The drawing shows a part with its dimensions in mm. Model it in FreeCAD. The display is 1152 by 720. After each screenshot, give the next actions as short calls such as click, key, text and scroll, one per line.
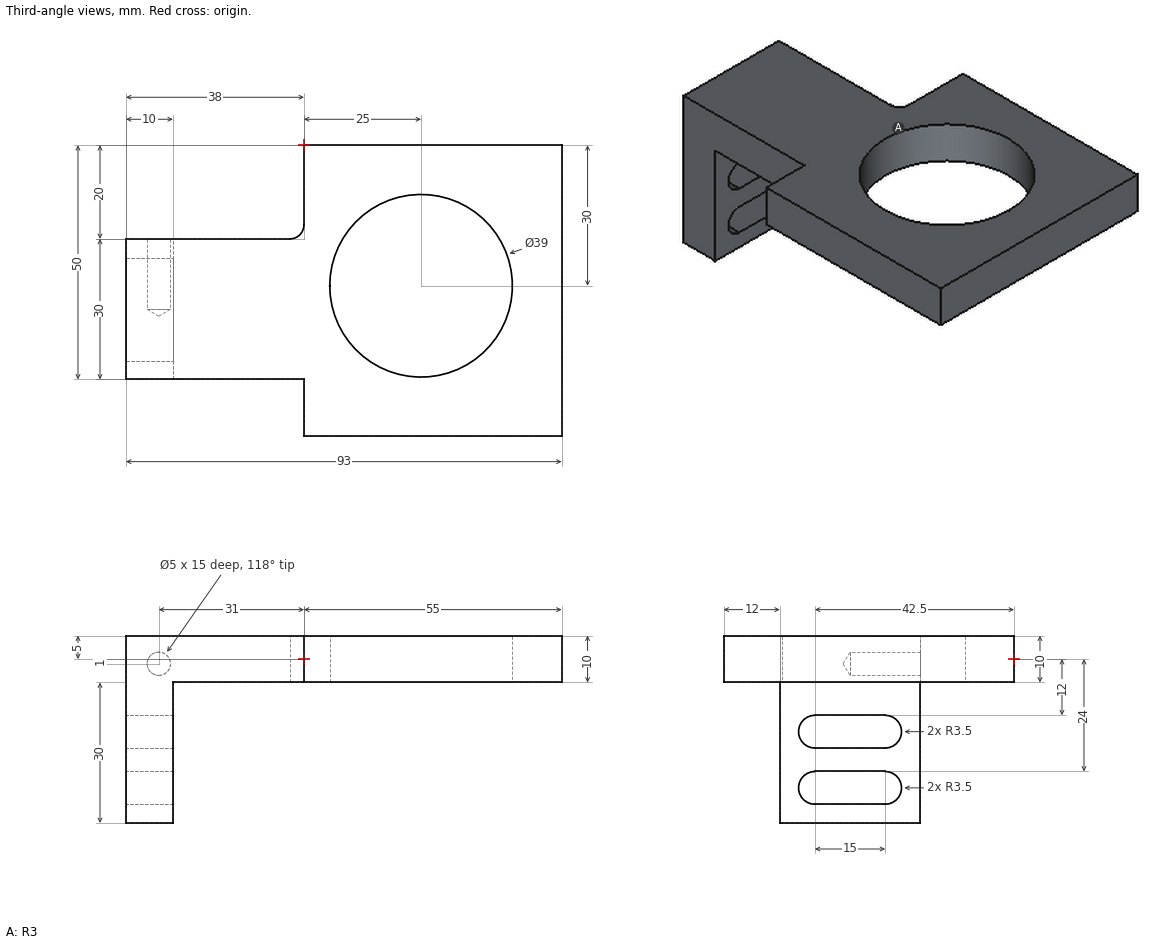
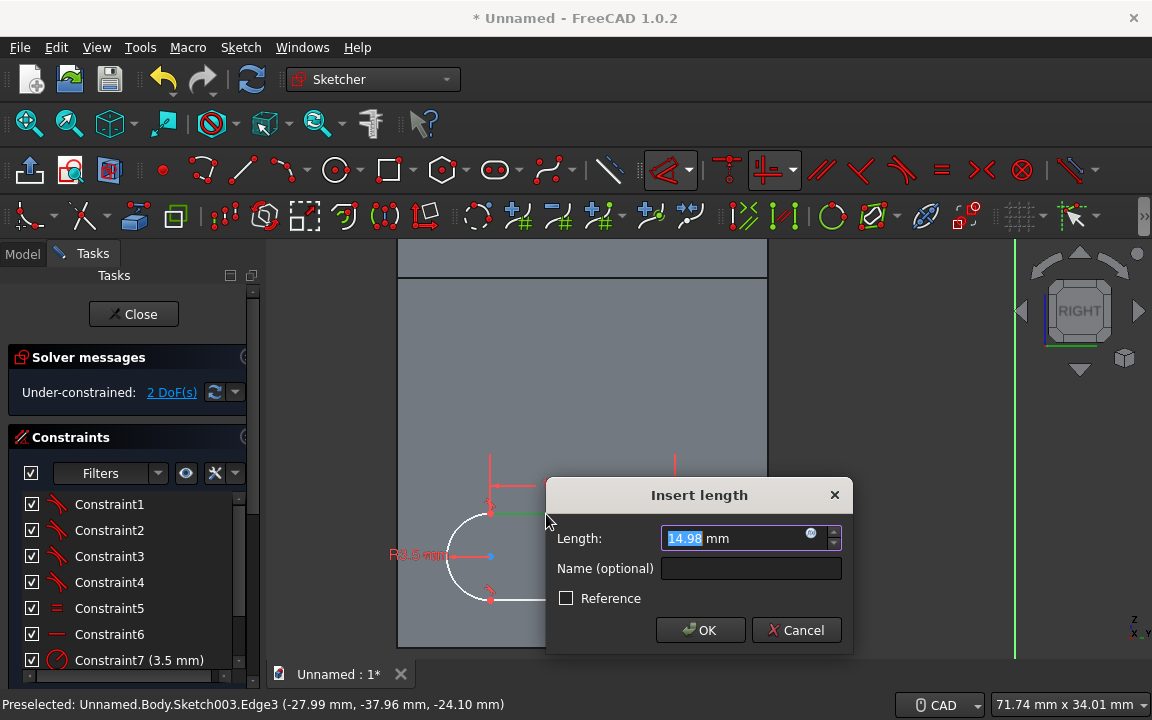
text(15)
key(Return)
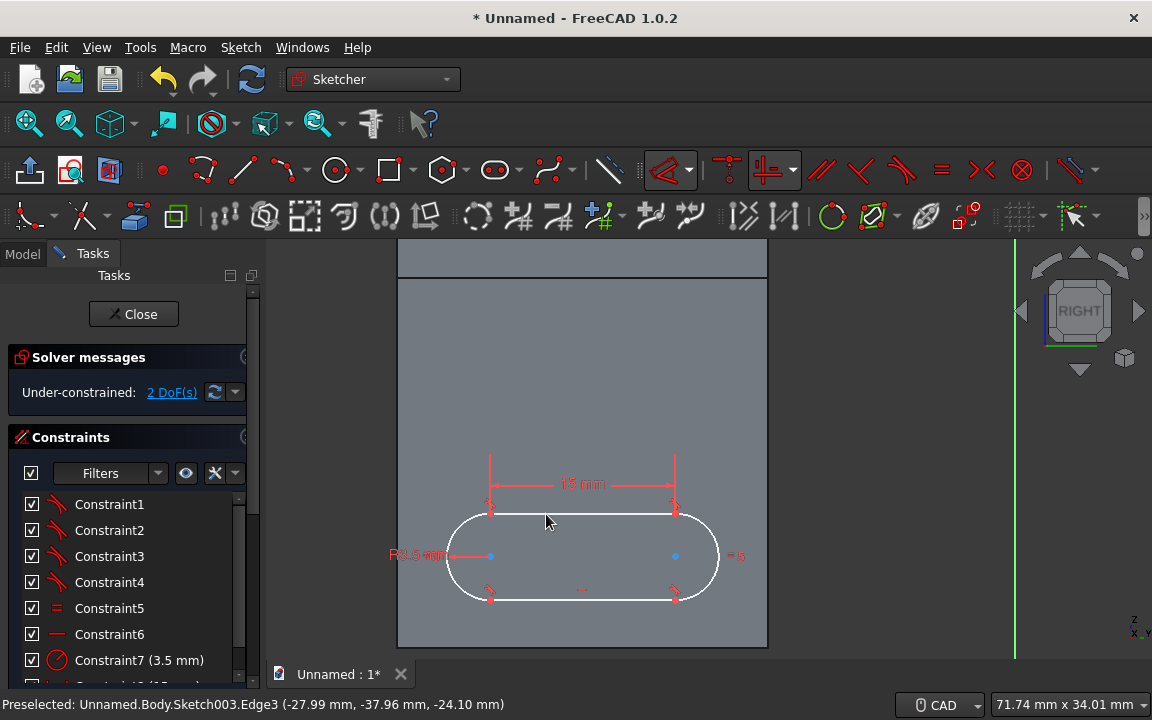
click(490, 514)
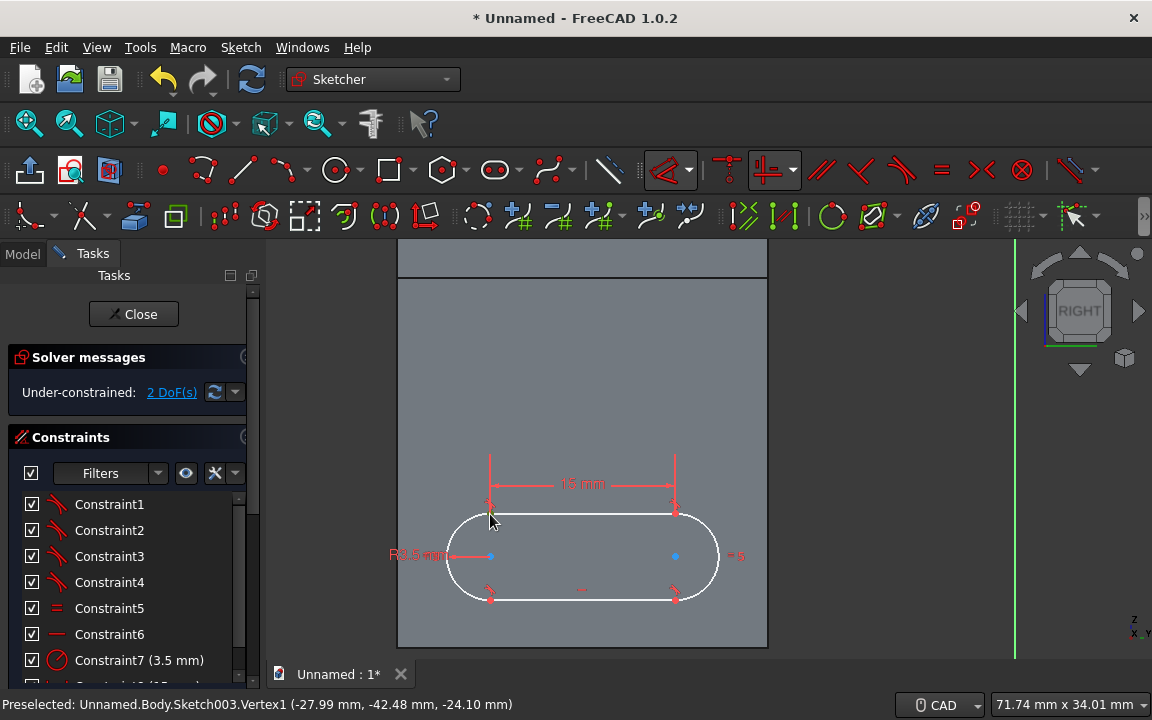
key(i)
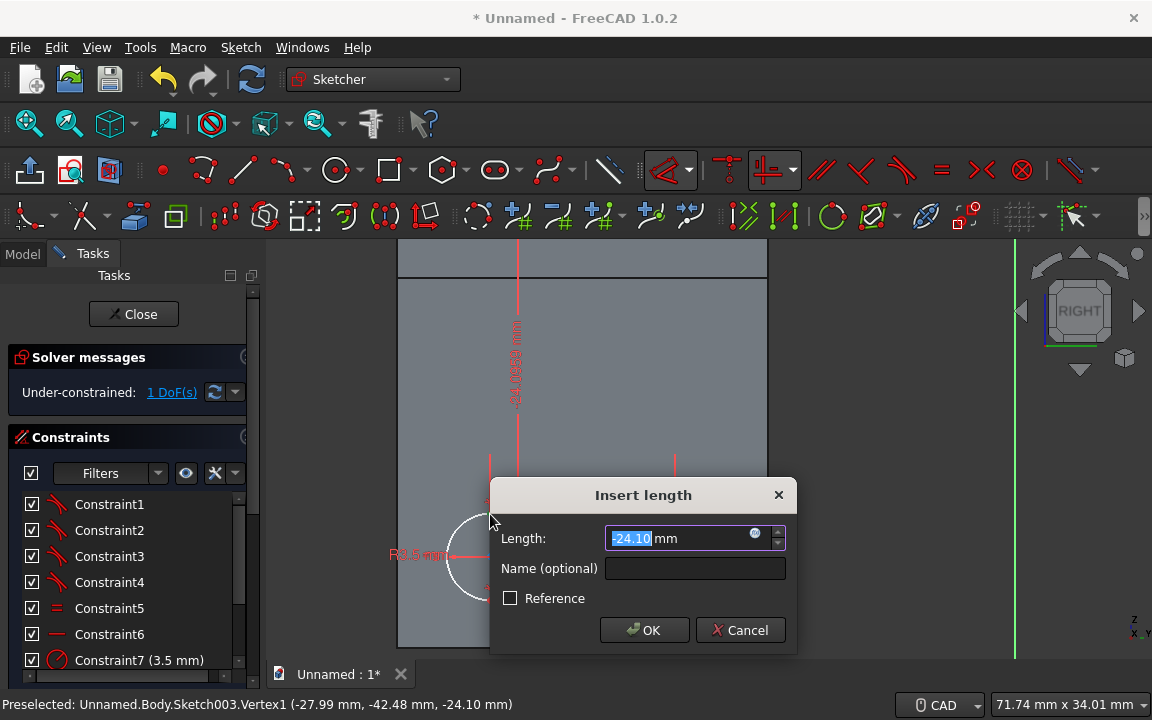
text(-24)
key(Return)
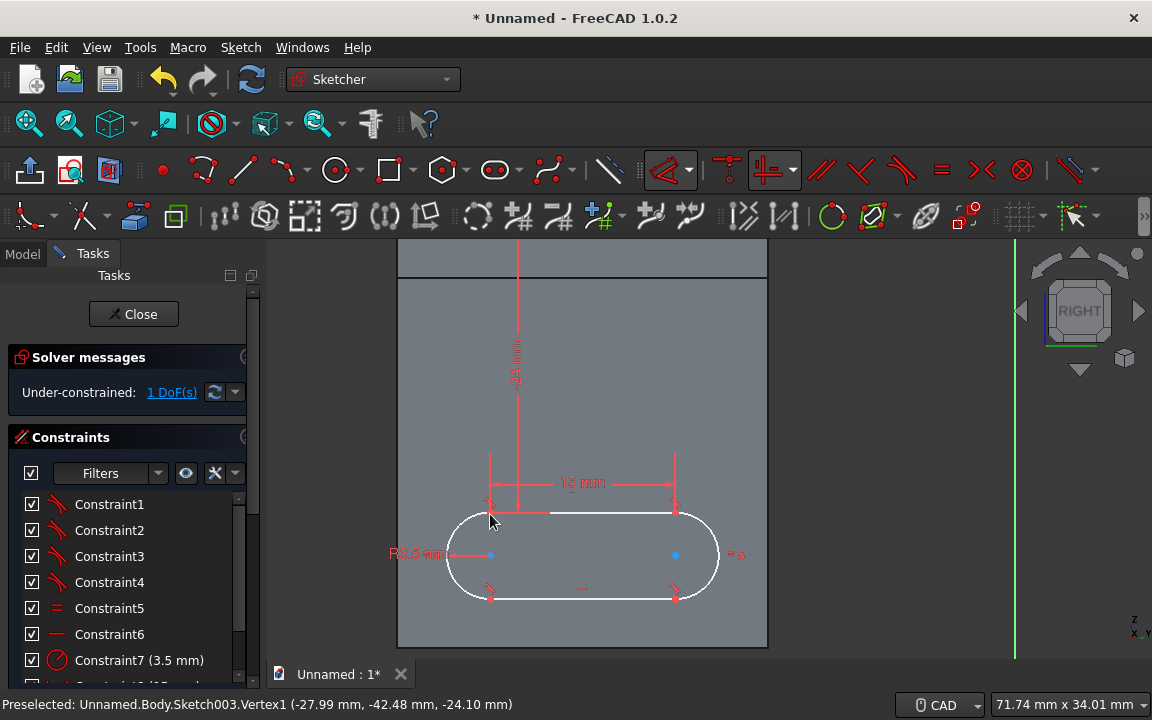
click(490, 513)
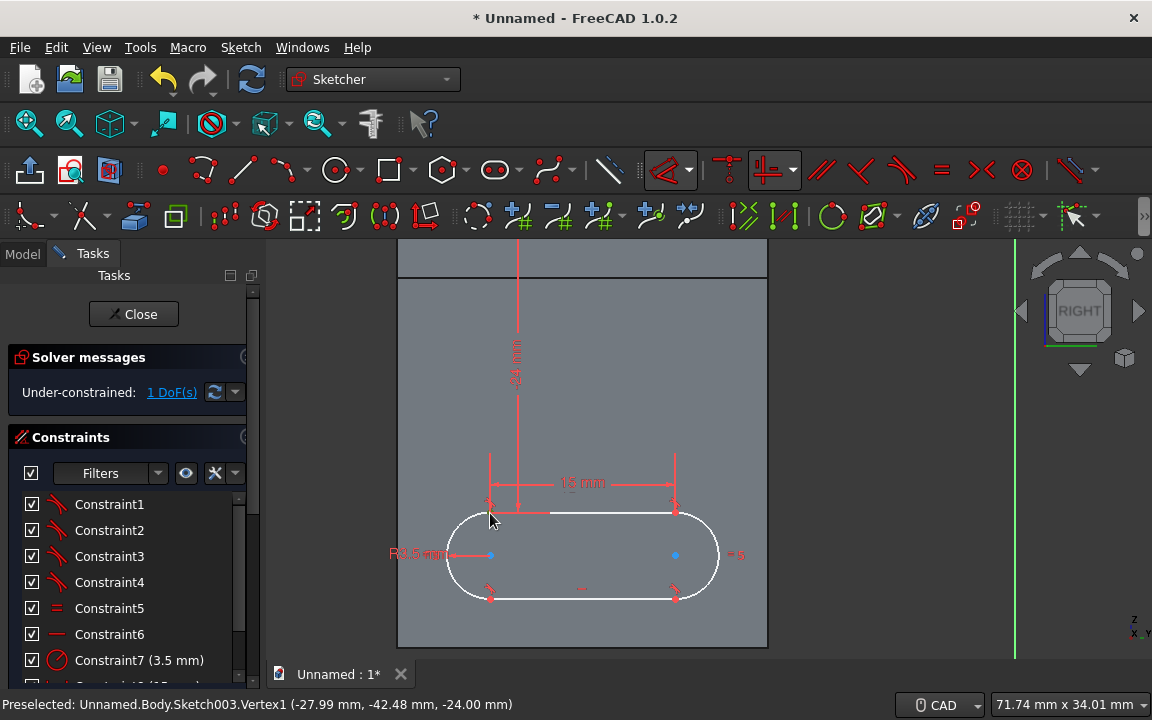
click(692, 170)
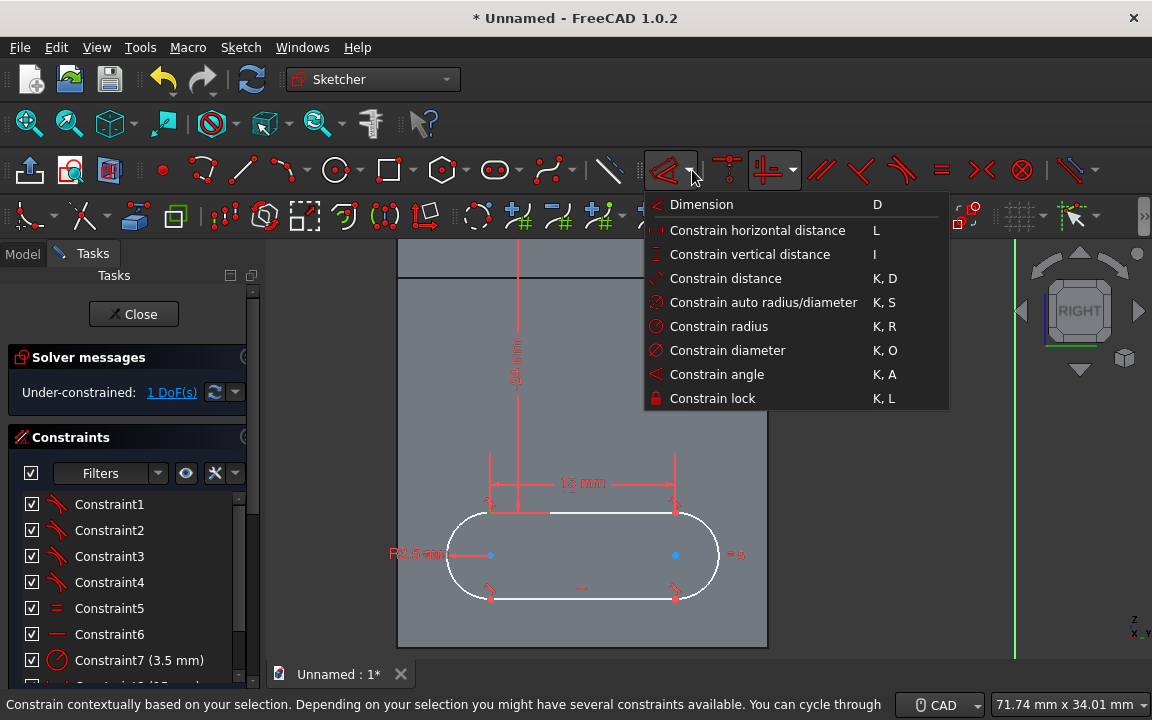
click(797, 230)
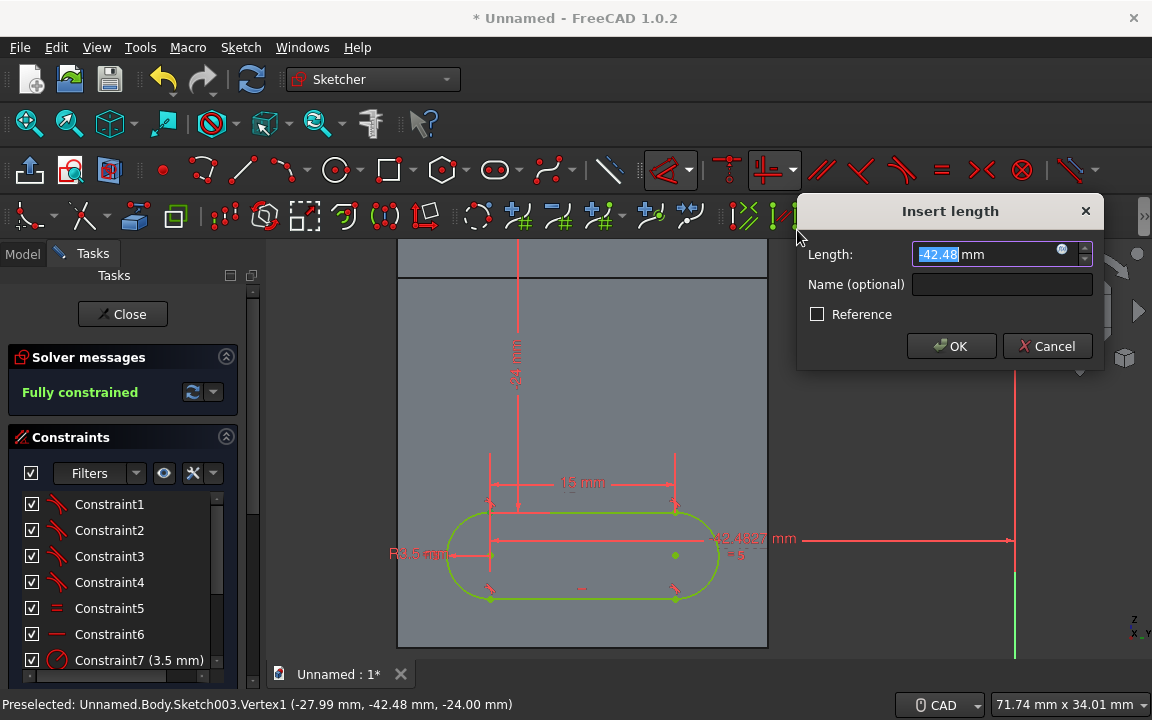
text(-42.5)
key(Return)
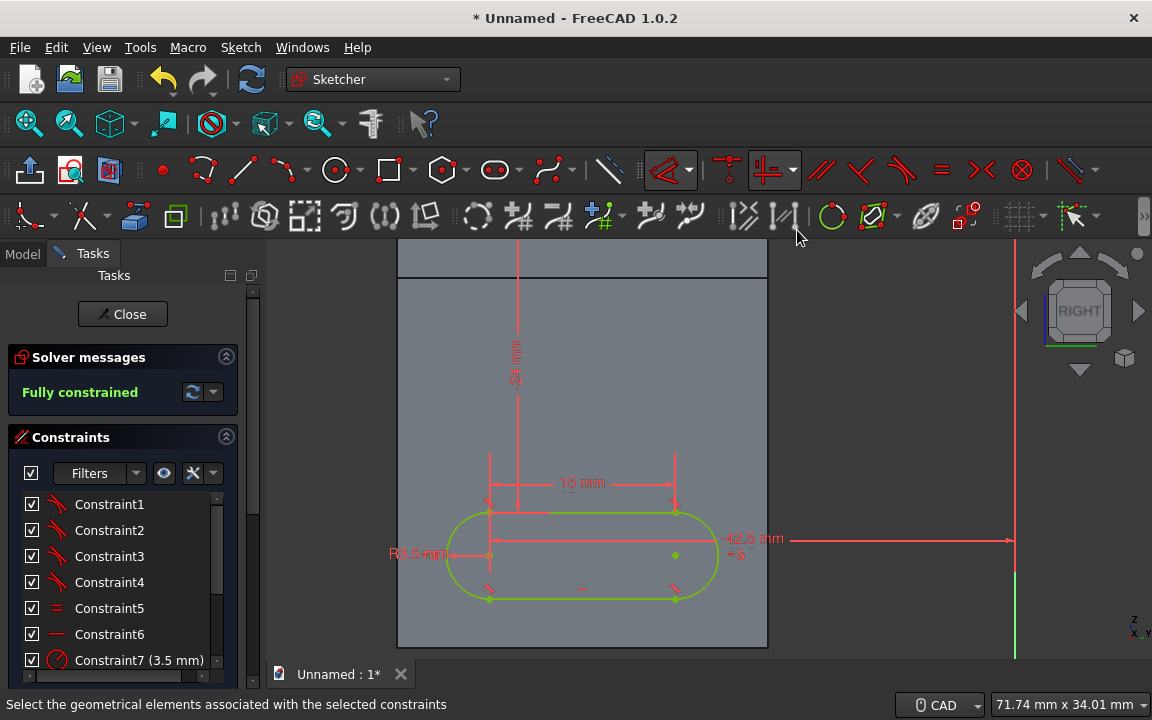
click(123, 314)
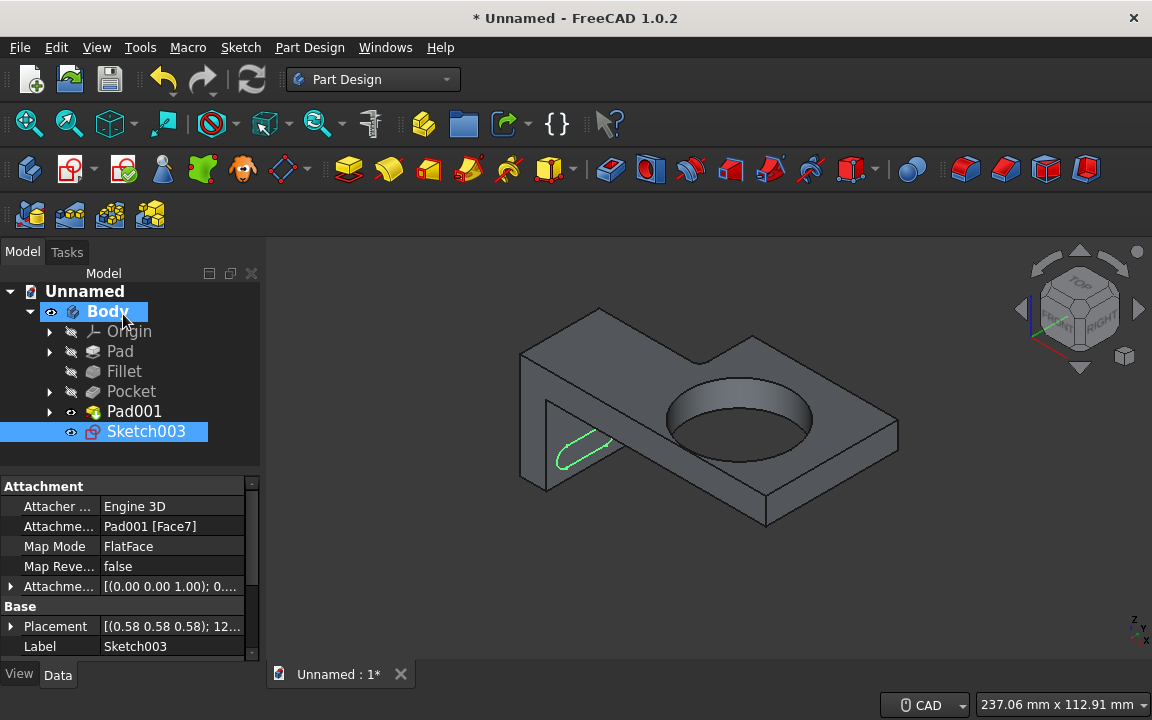
click(612, 170)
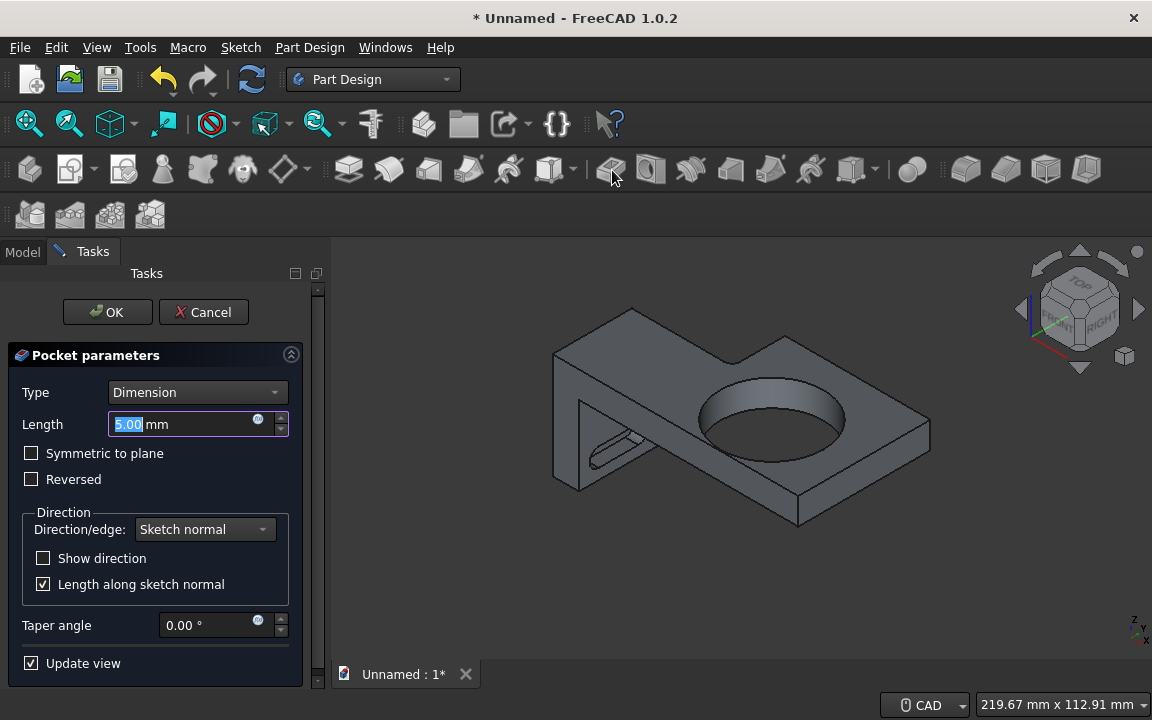
click(198, 392)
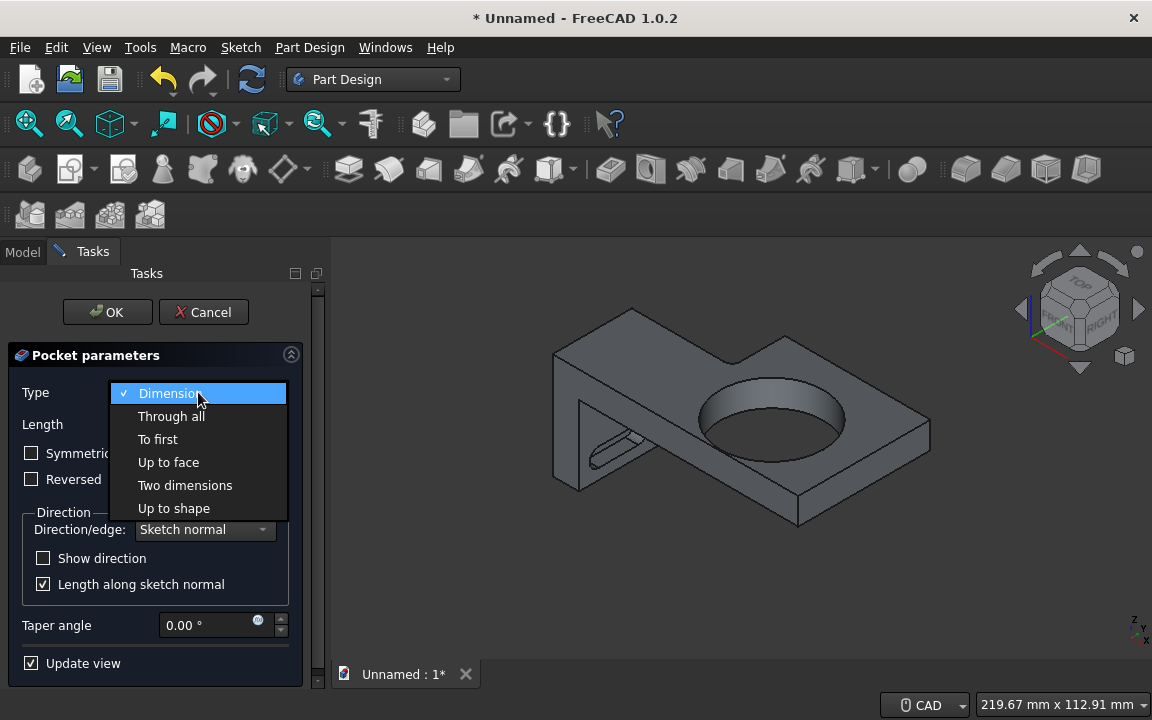
click(198, 440)